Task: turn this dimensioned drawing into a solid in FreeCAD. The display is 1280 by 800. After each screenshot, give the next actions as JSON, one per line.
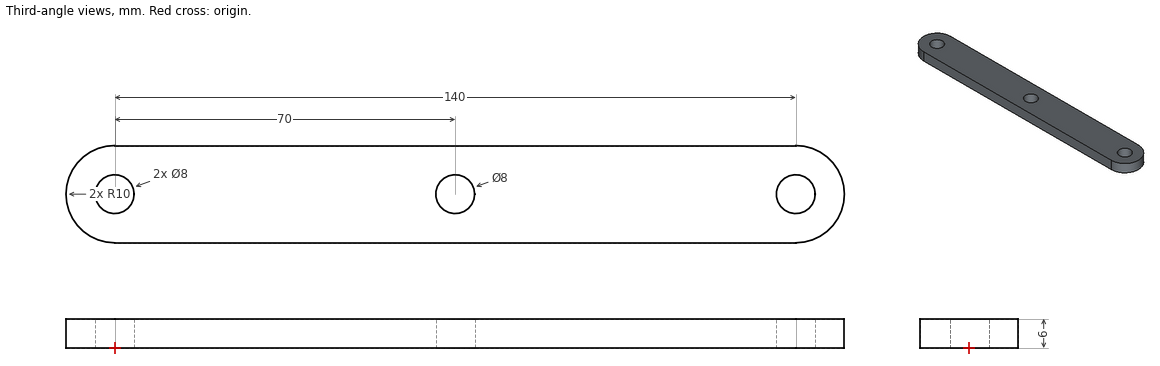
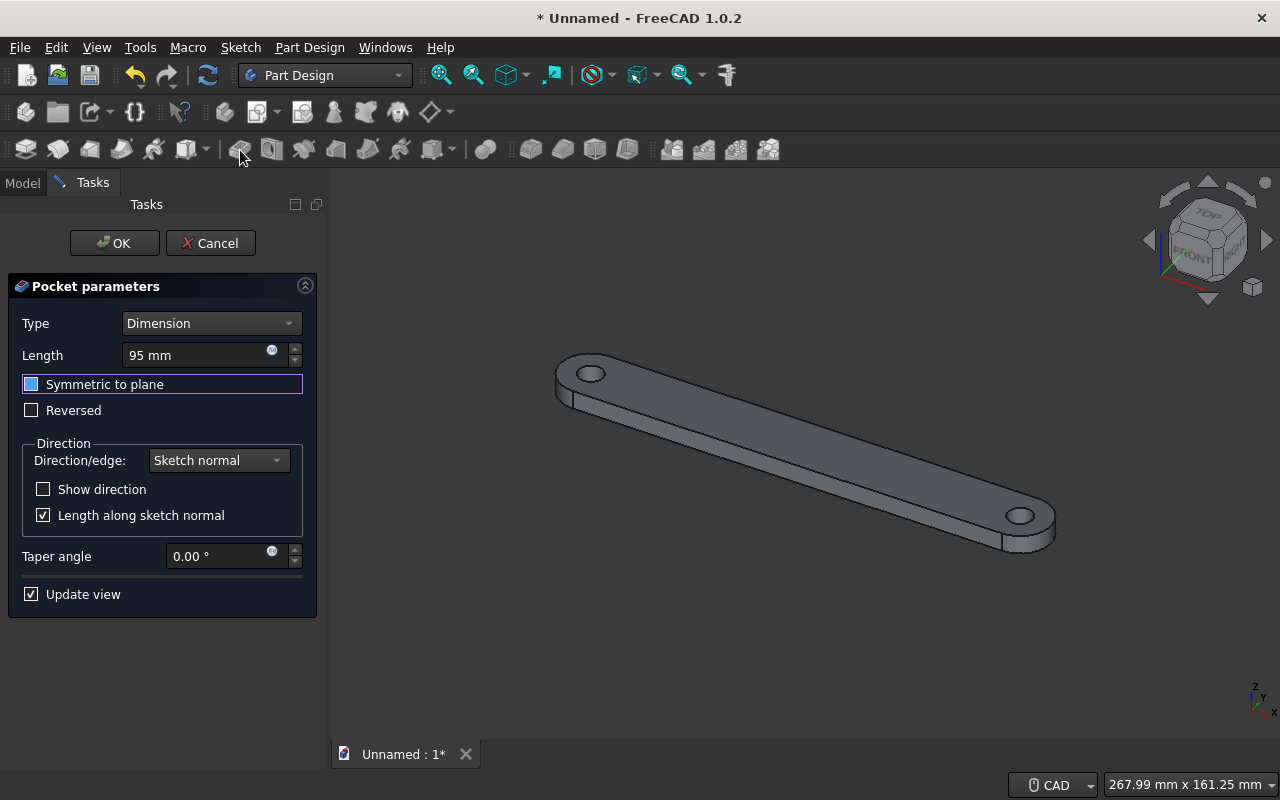
{"action": "left_click", "coordinate": [115, 243]}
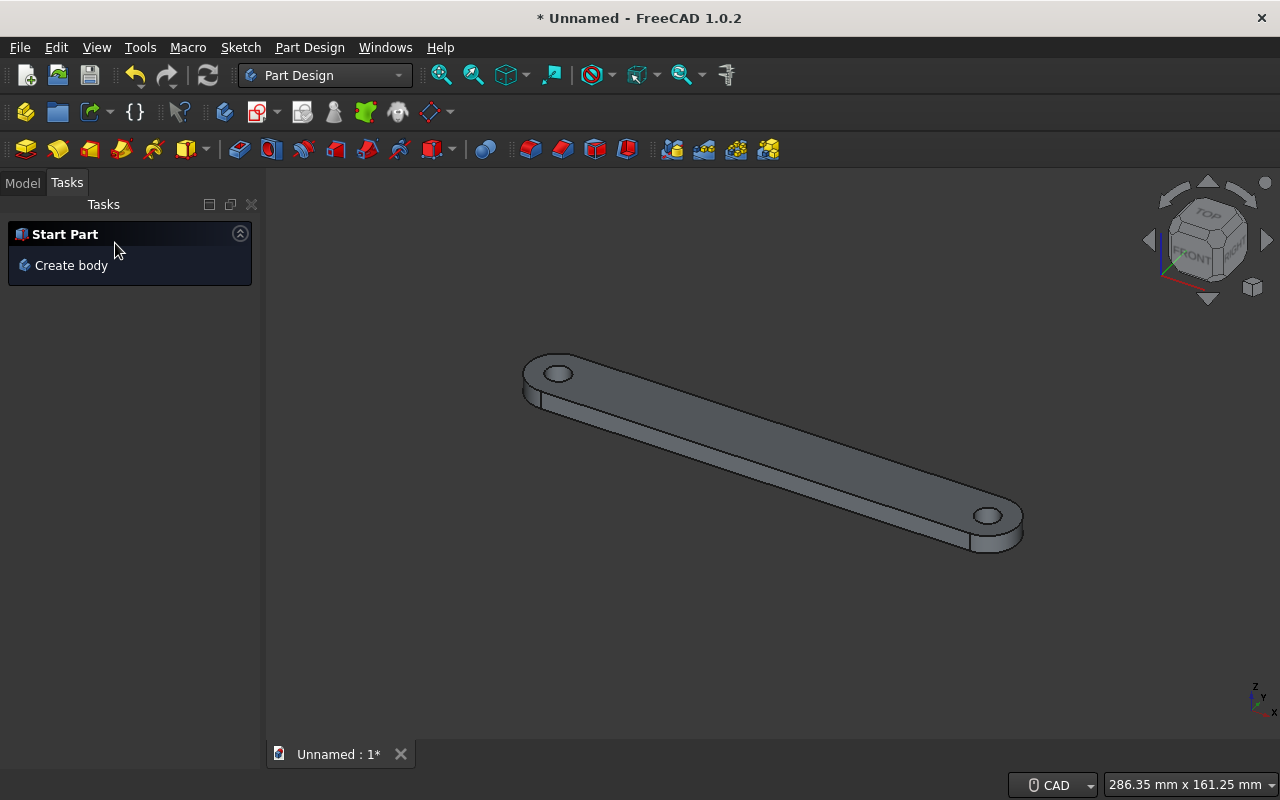
{"action": "left_click", "coordinate": [913, 490]}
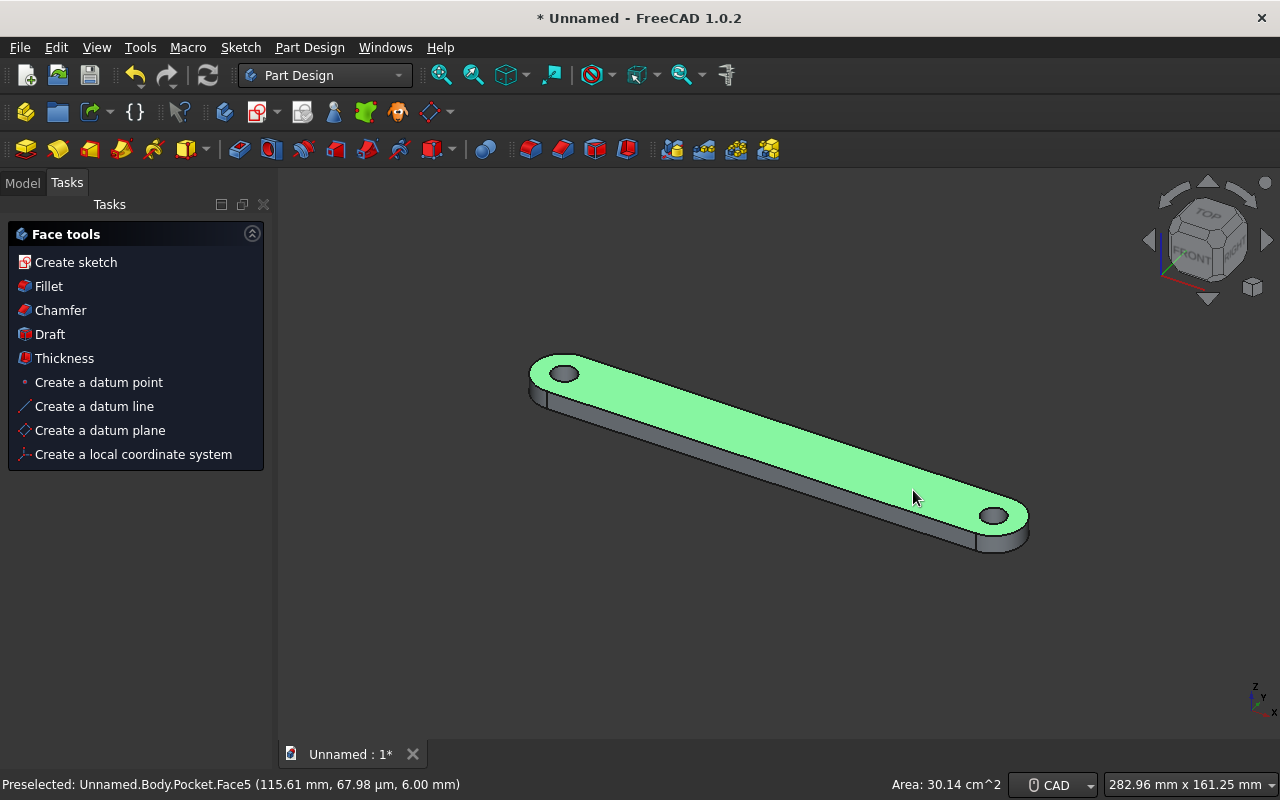
{"action": "left_click", "coordinate": [258, 112]}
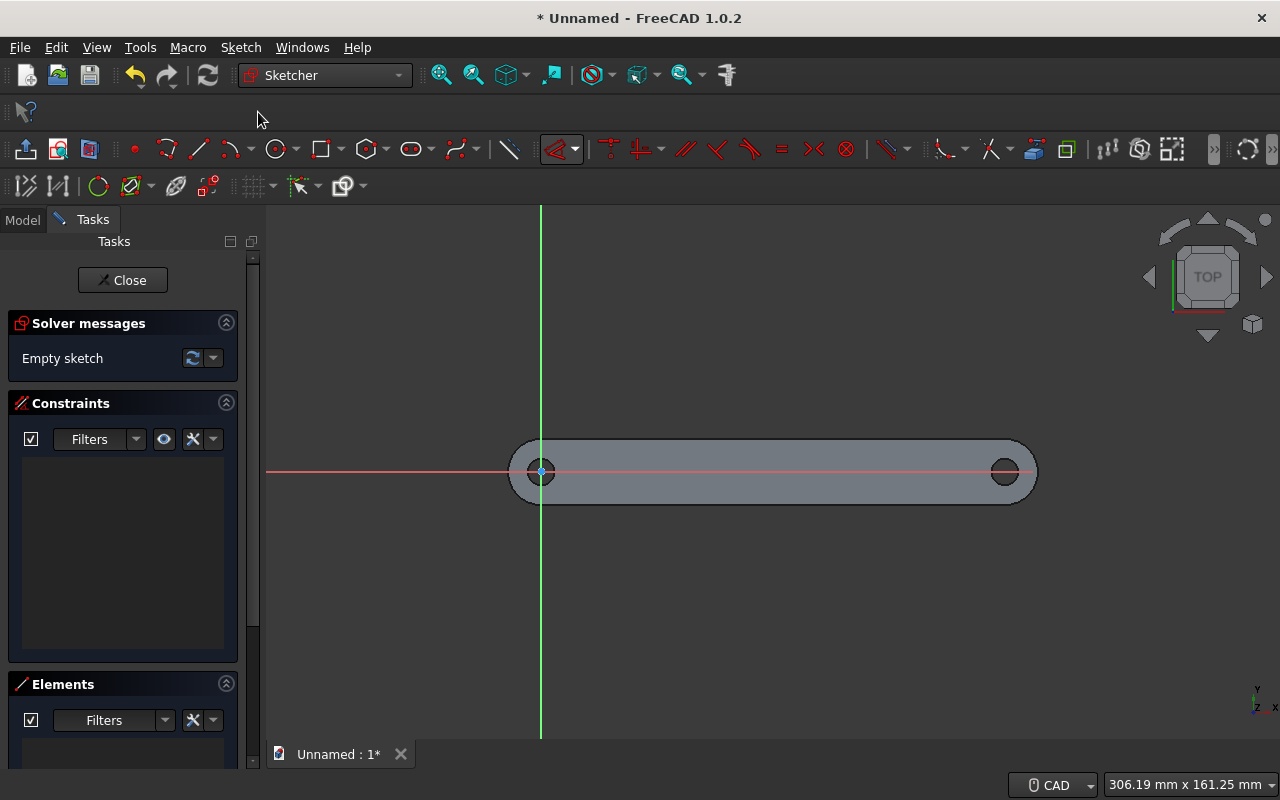
{"action": "scroll", "coordinate": [778, 472], "scroll_direction": "up", "scroll_amount": 13}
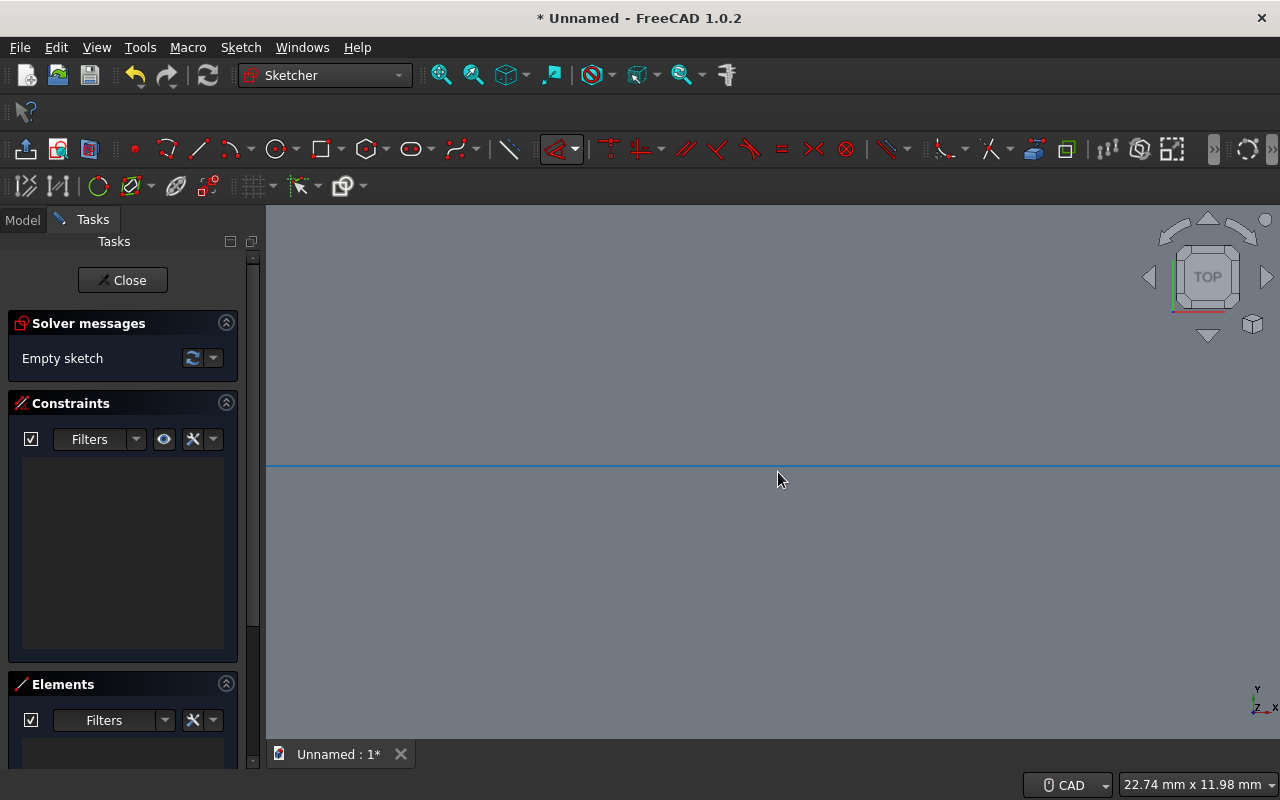
{"action": "key", "text": "g c"}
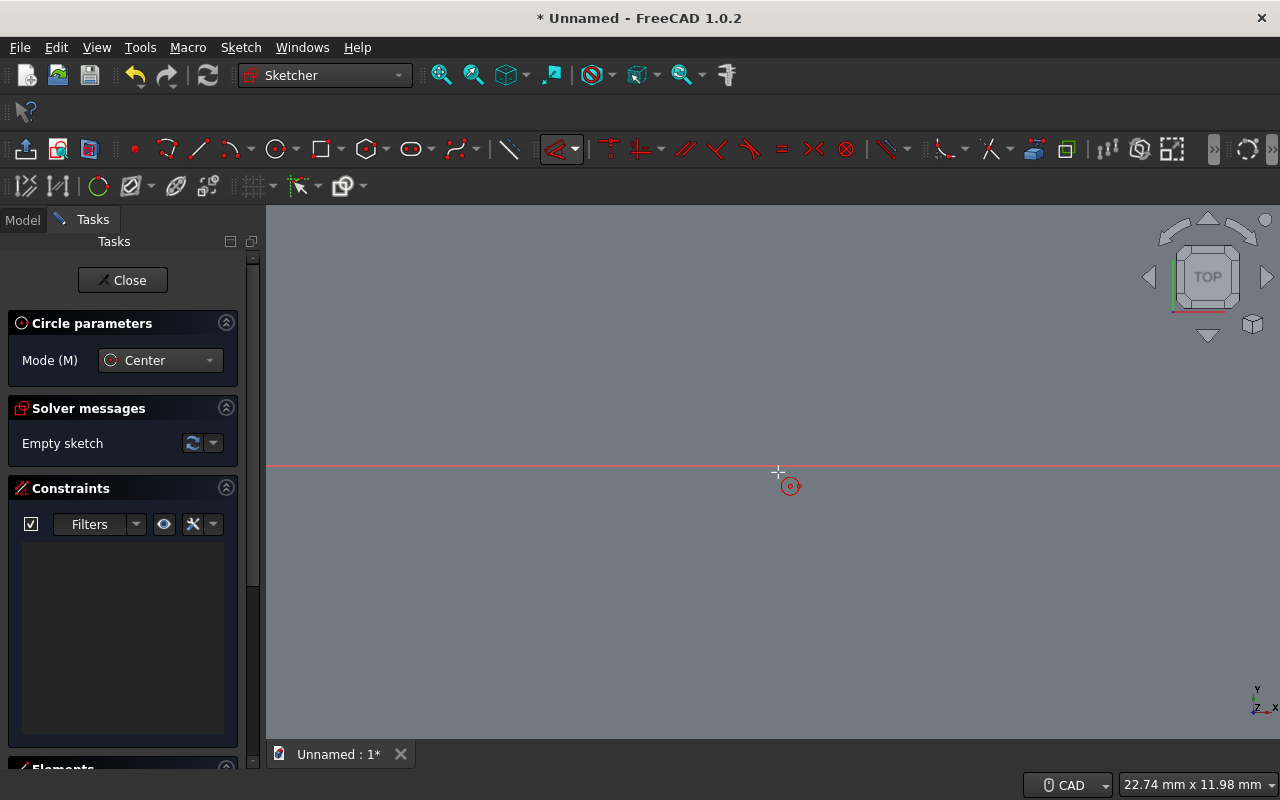
{"action": "left_click", "coordinate": [704, 466]}
{"action": "left_click", "coordinate": [830, 340]}
{"action": "key", "text": "Escape"}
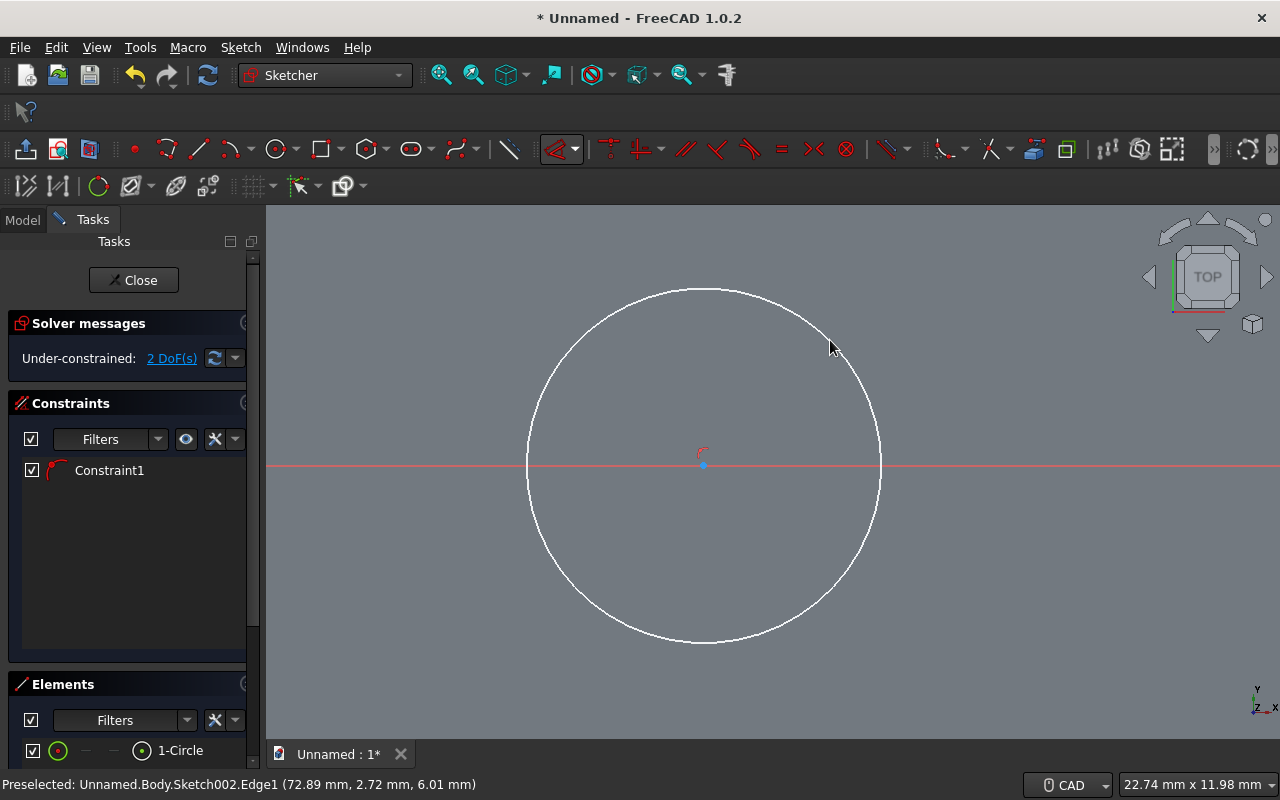
{"action": "left_click", "coordinate": [829, 340]}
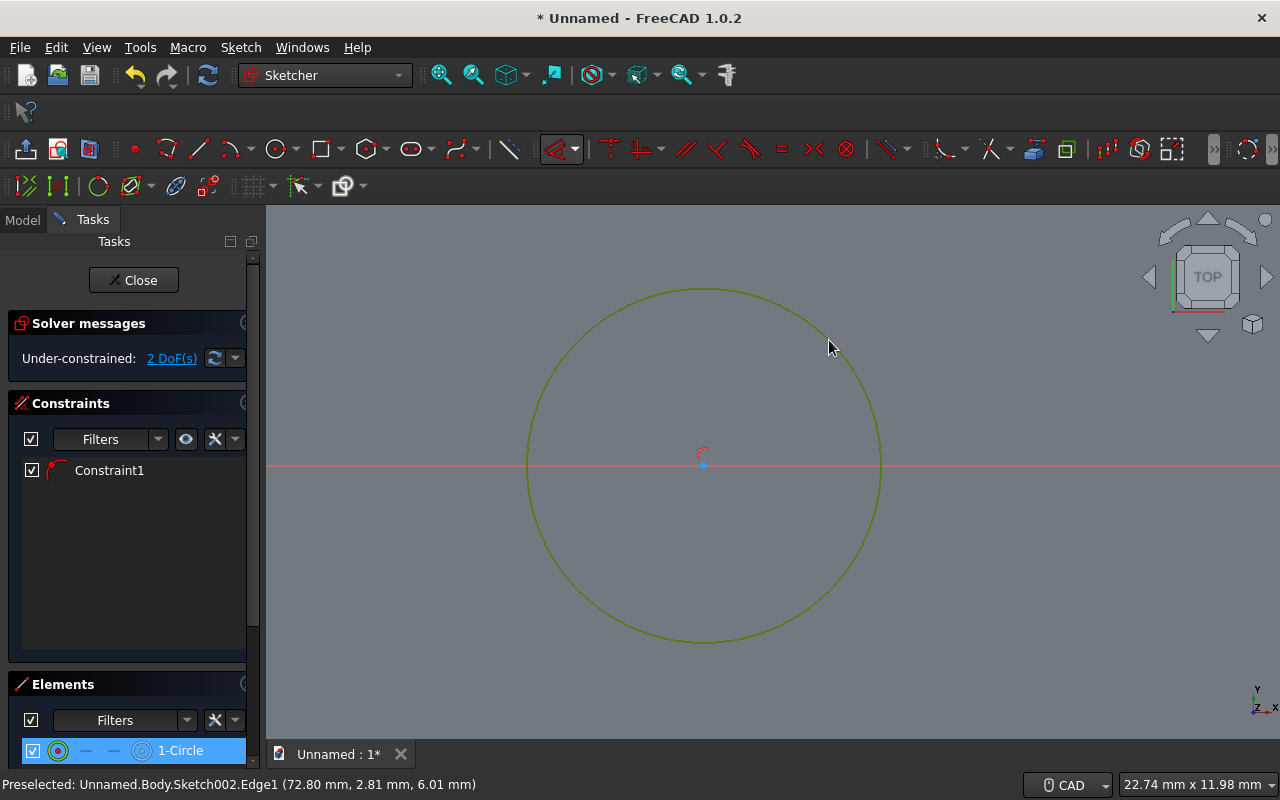
{"action": "left_click", "coordinate": [578, 150]}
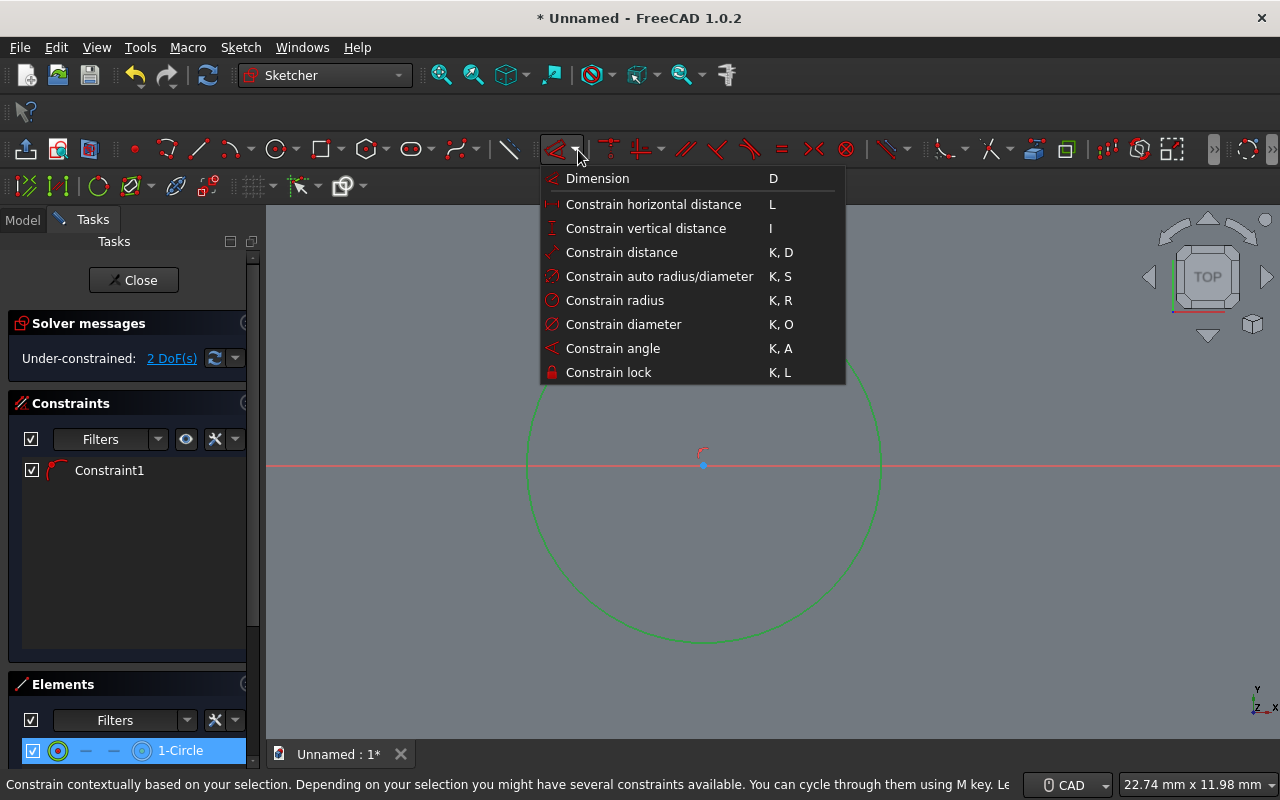
{"action": "left_click", "coordinate": [693, 324]}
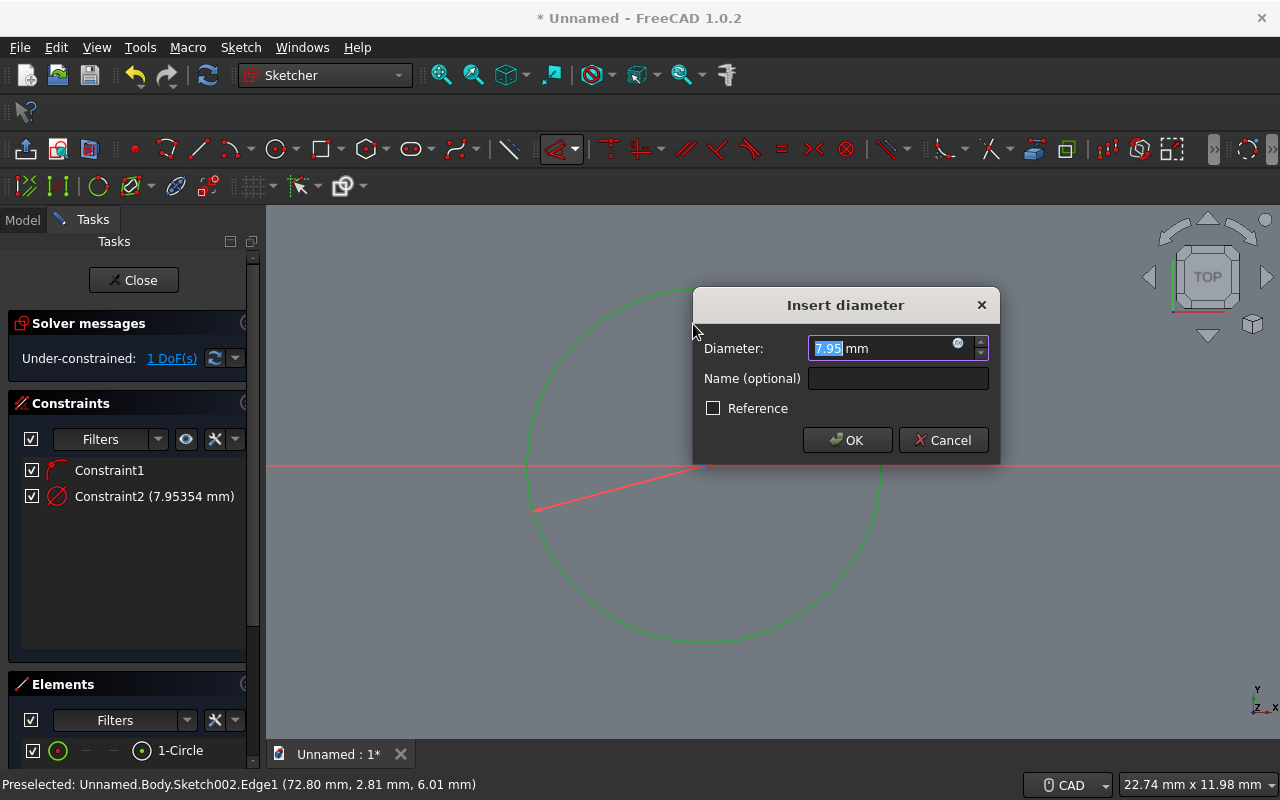
{"action": "type", "text": "8"}
{"action": "key", "text": "Return"}